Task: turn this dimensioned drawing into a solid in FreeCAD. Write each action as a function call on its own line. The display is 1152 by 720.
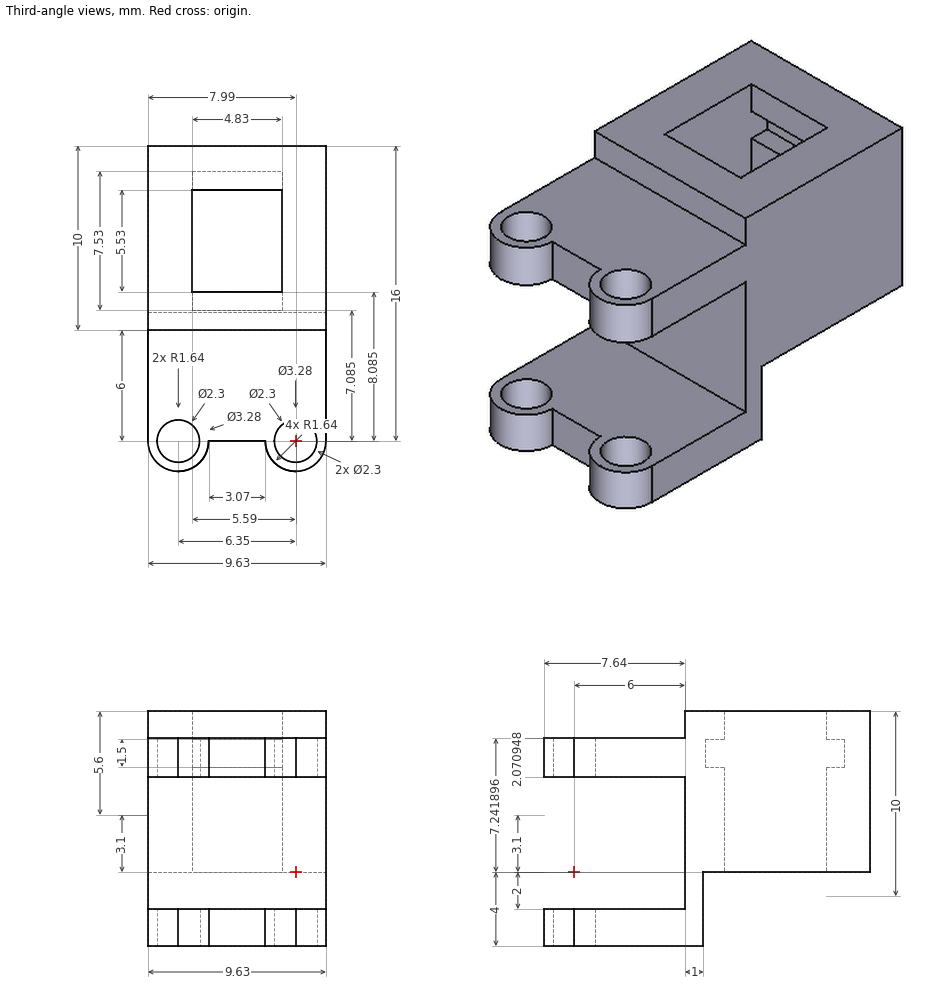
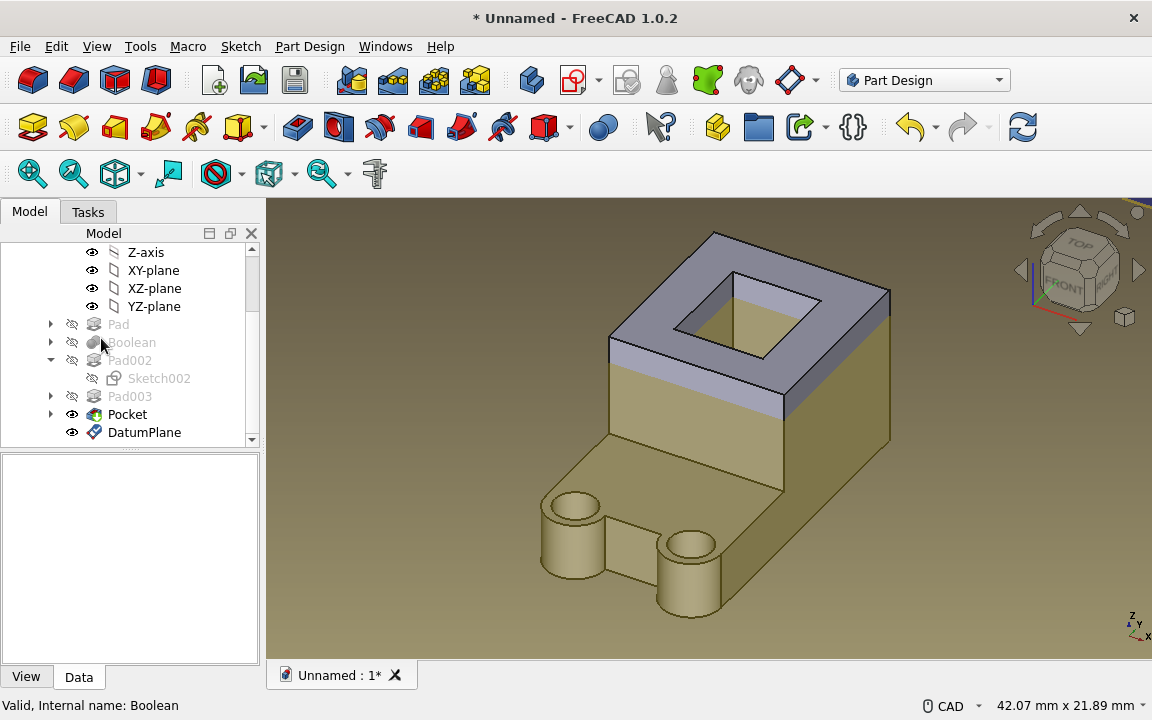
click(117, 432)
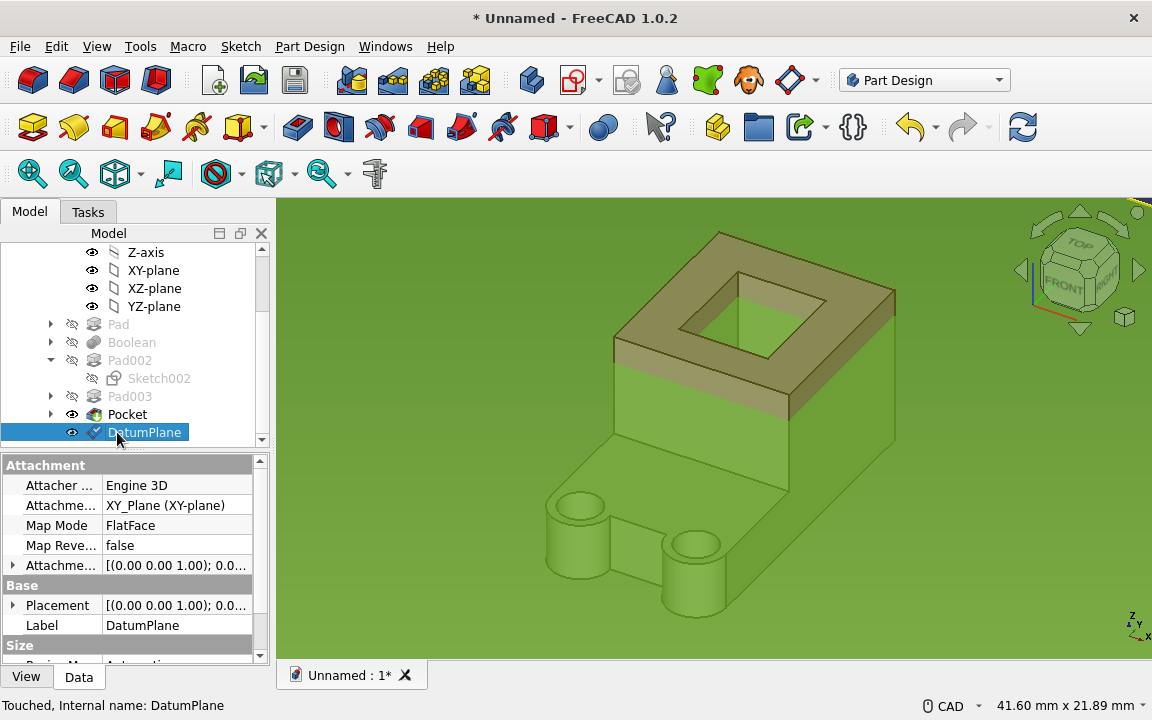
click(572, 80)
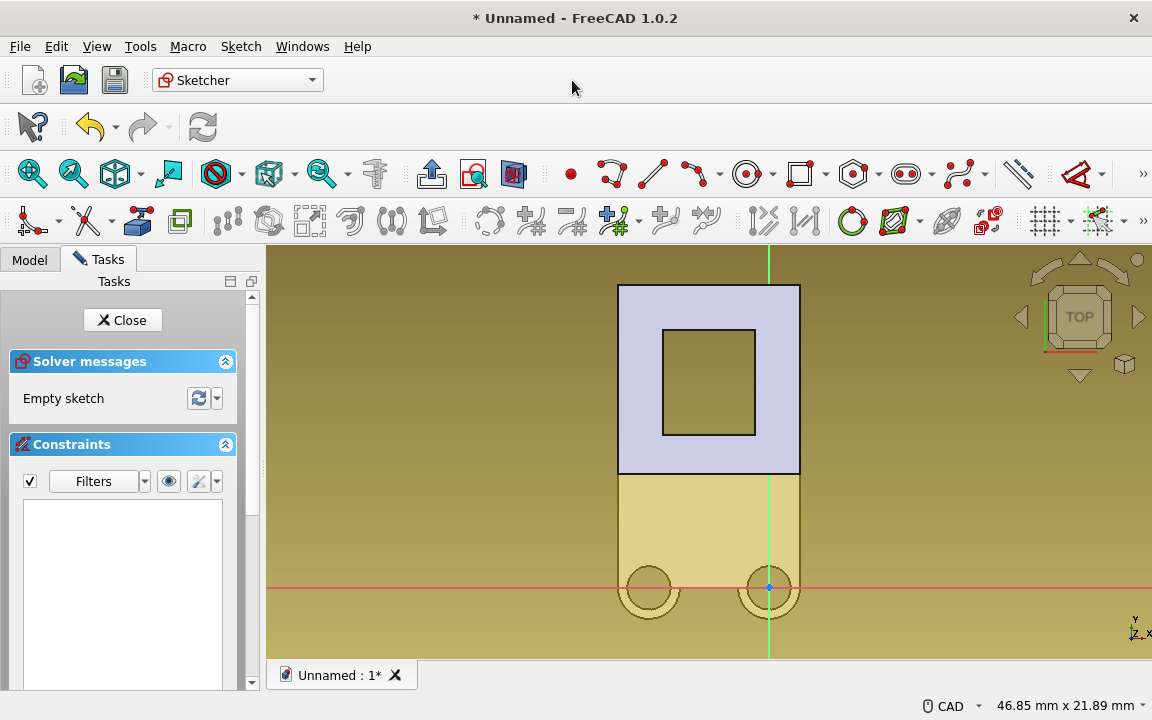
click(514, 174)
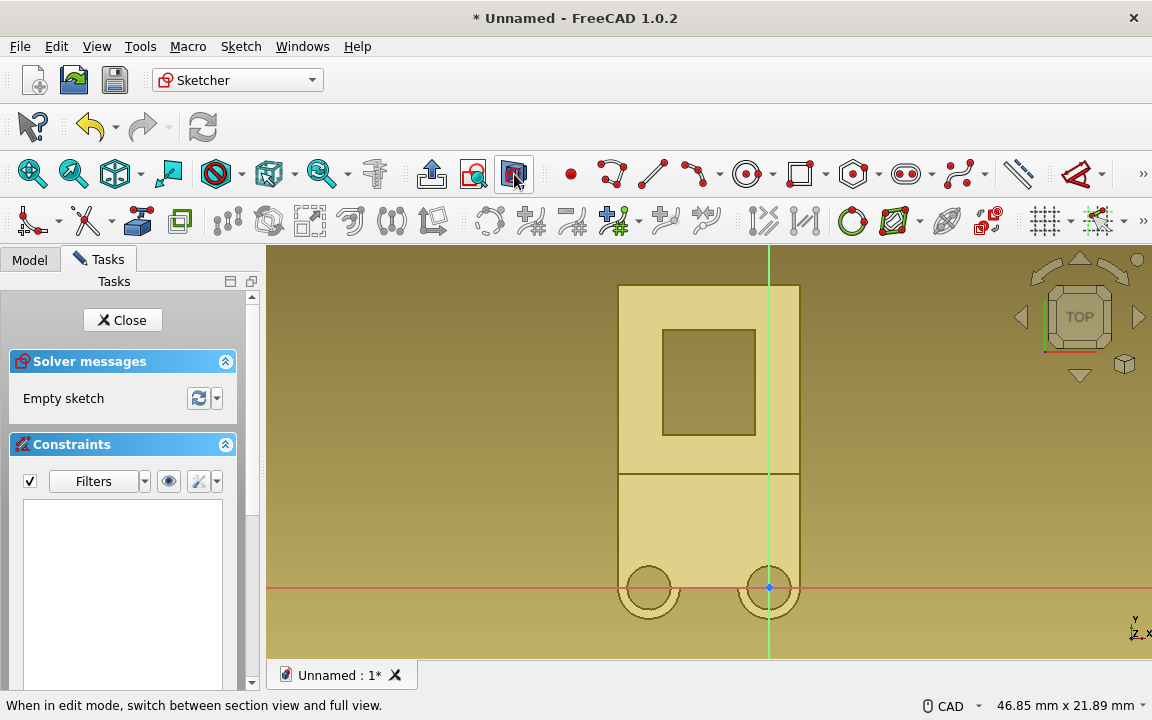
key(g)
key(r)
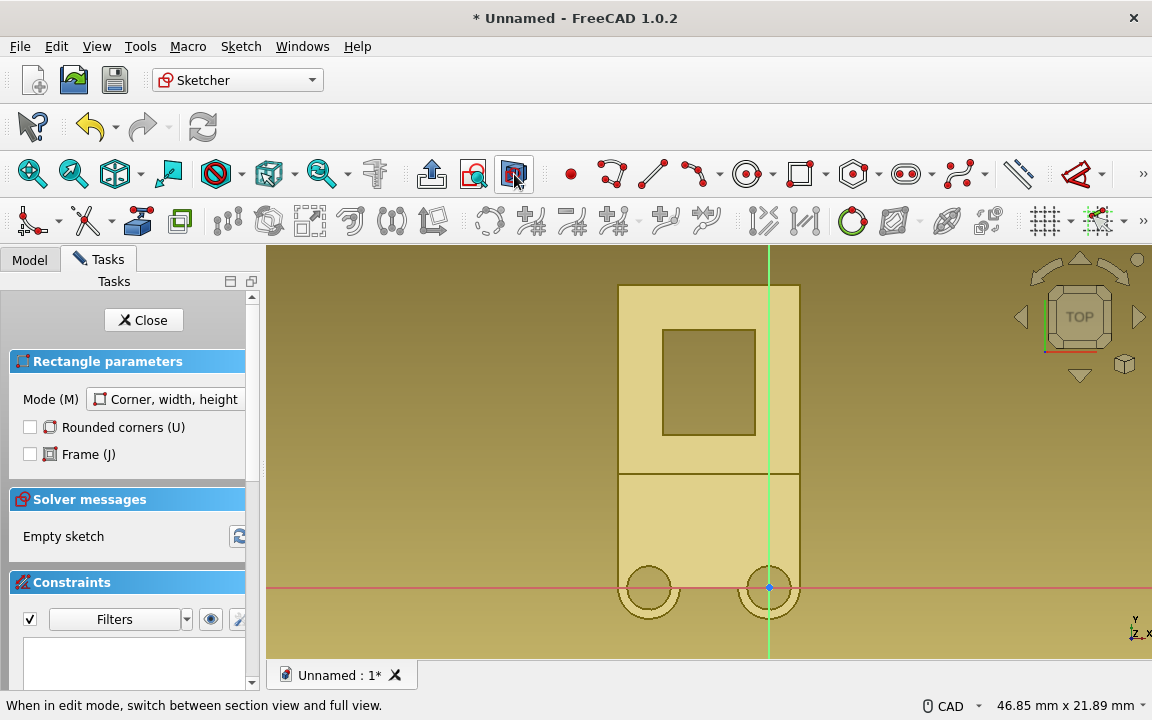
click(663, 311)
click(755, 454)
key(Escape)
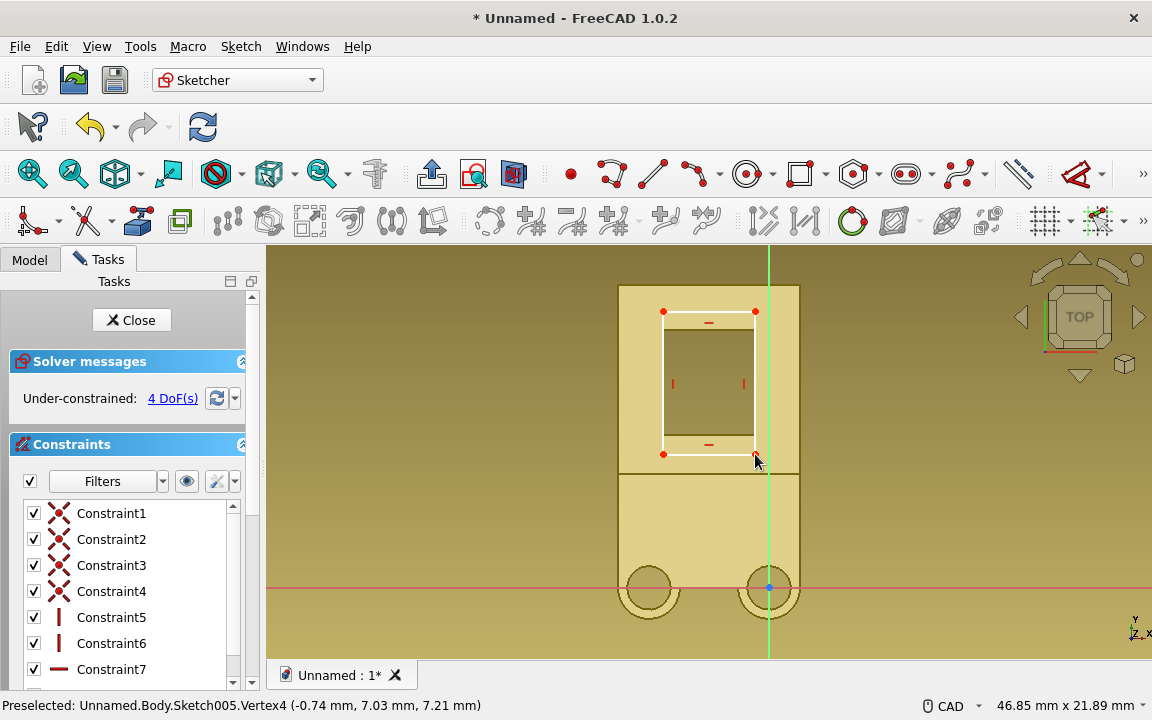
click(1076, 174)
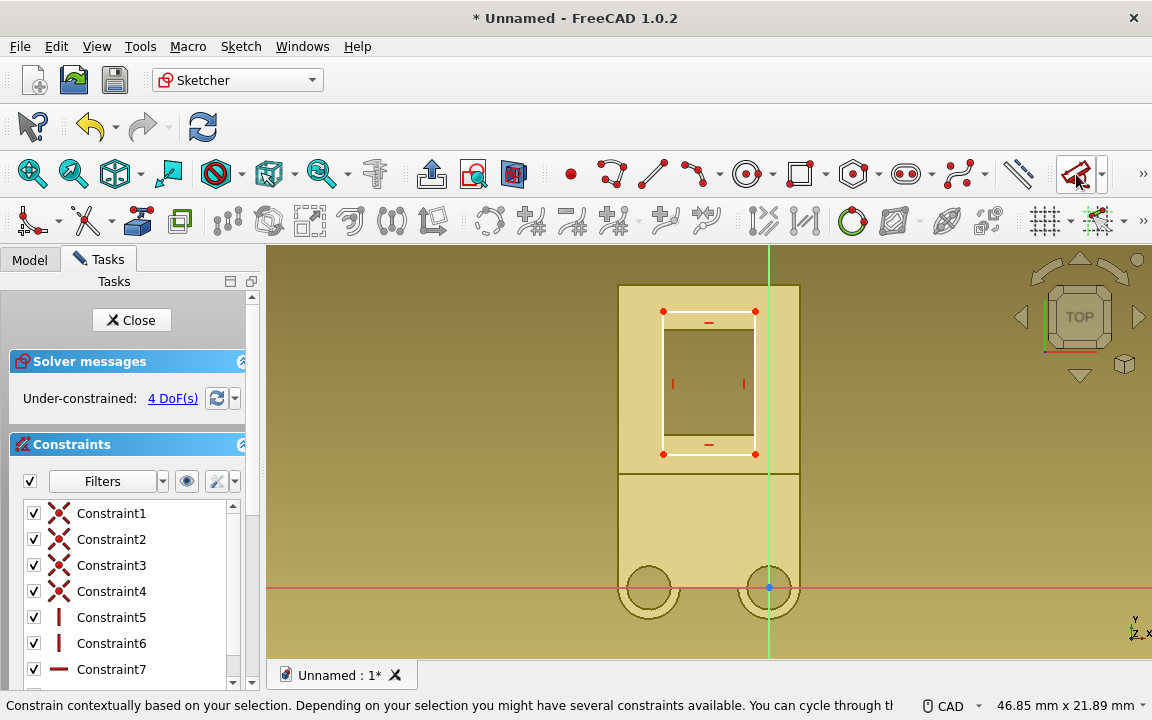
click(663, 355)
click(629, 384)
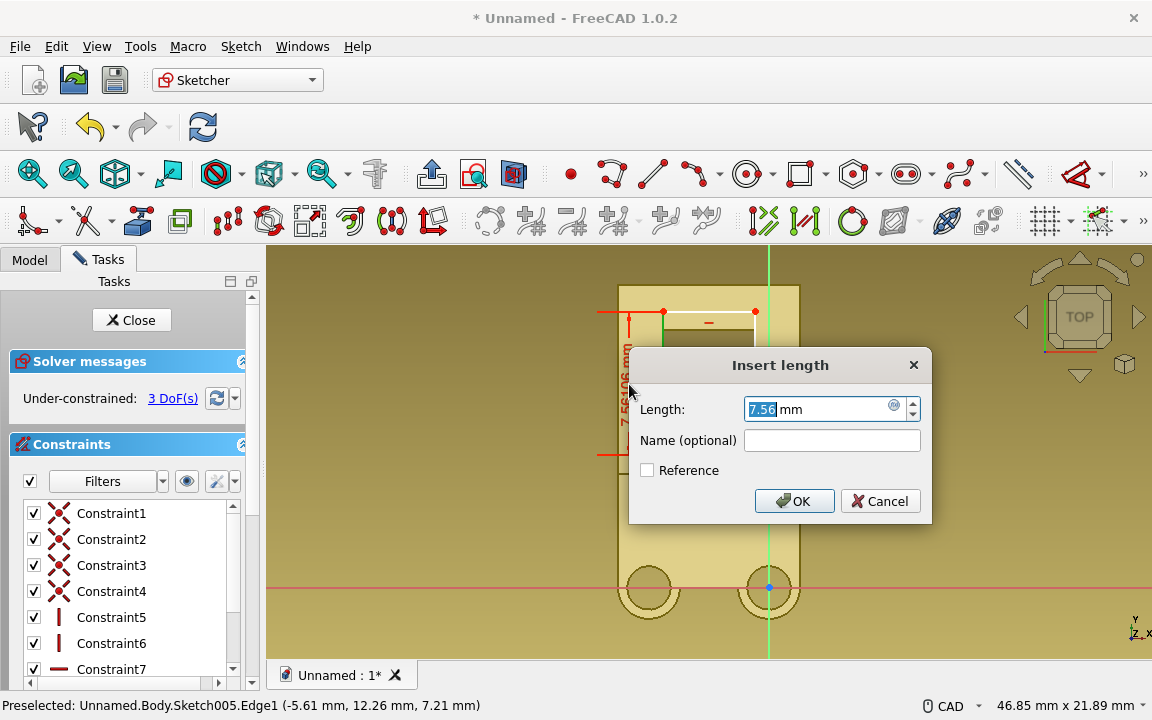
text(7.53)
key(Return)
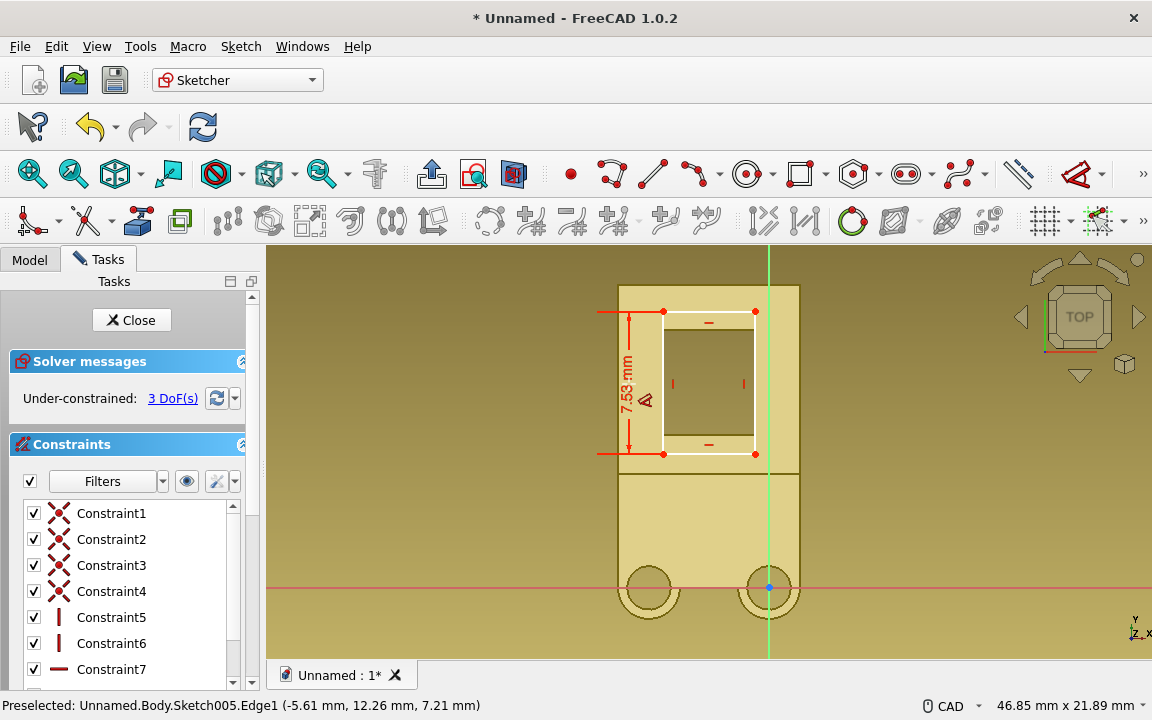
click(691, 454)
click(709, 488)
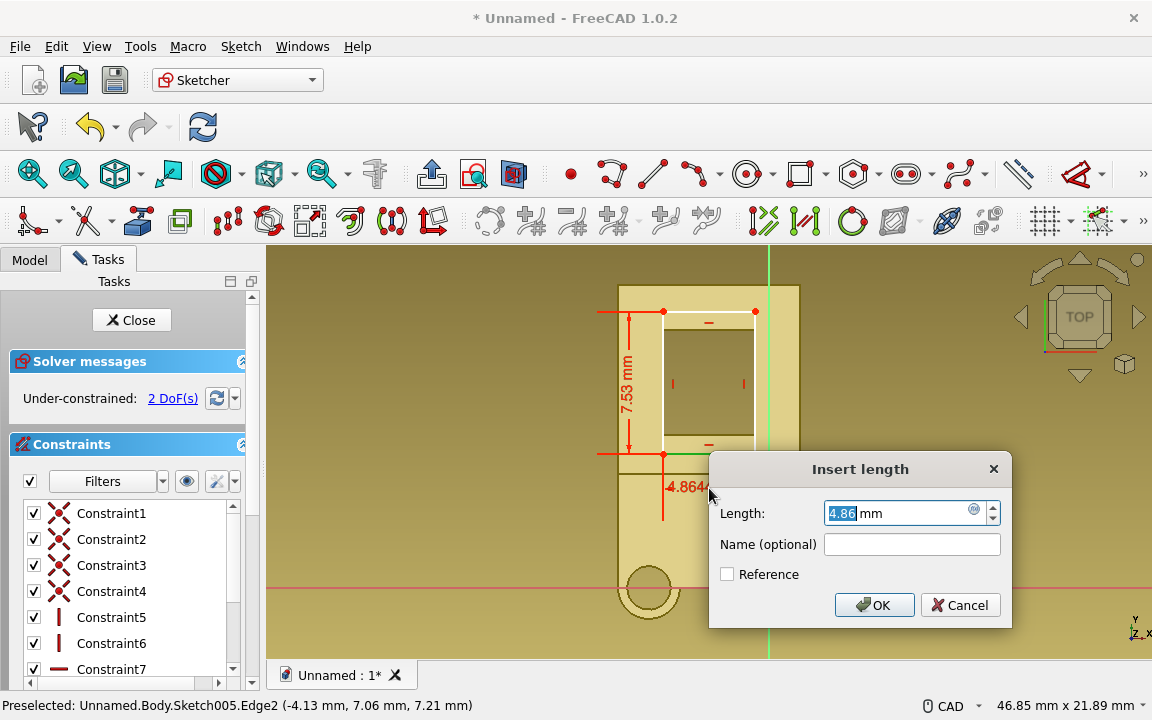
text(4.83)
key(Return)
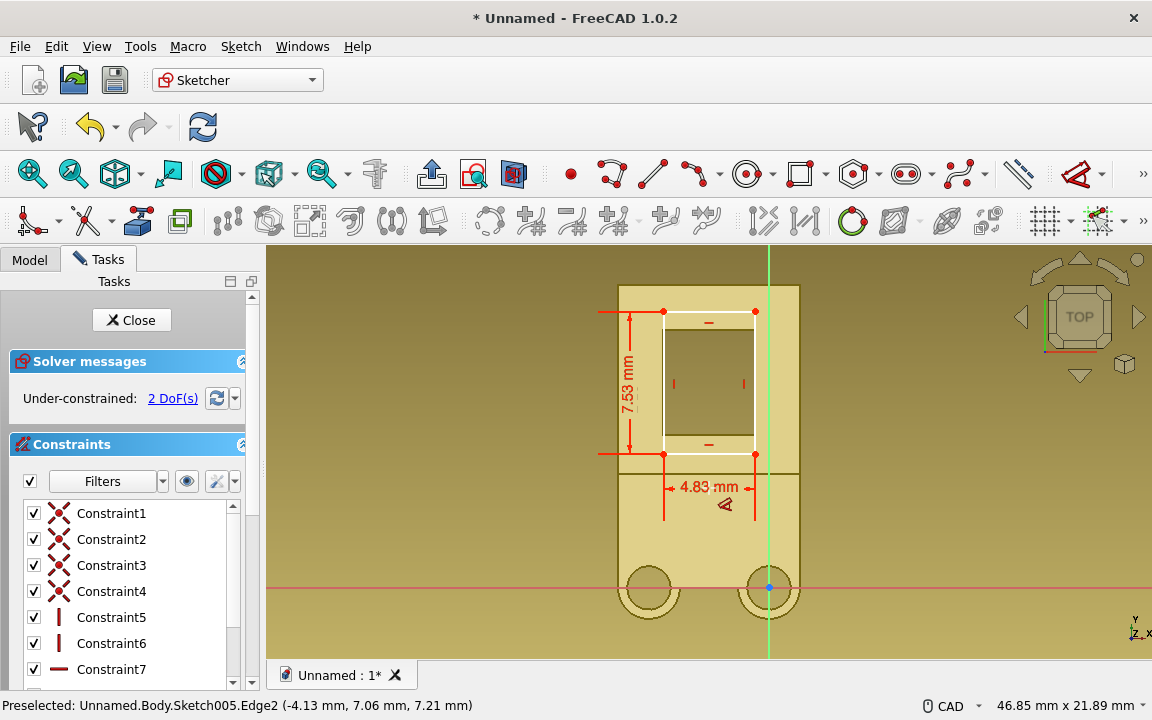
click(664, 312)
click(716, 622)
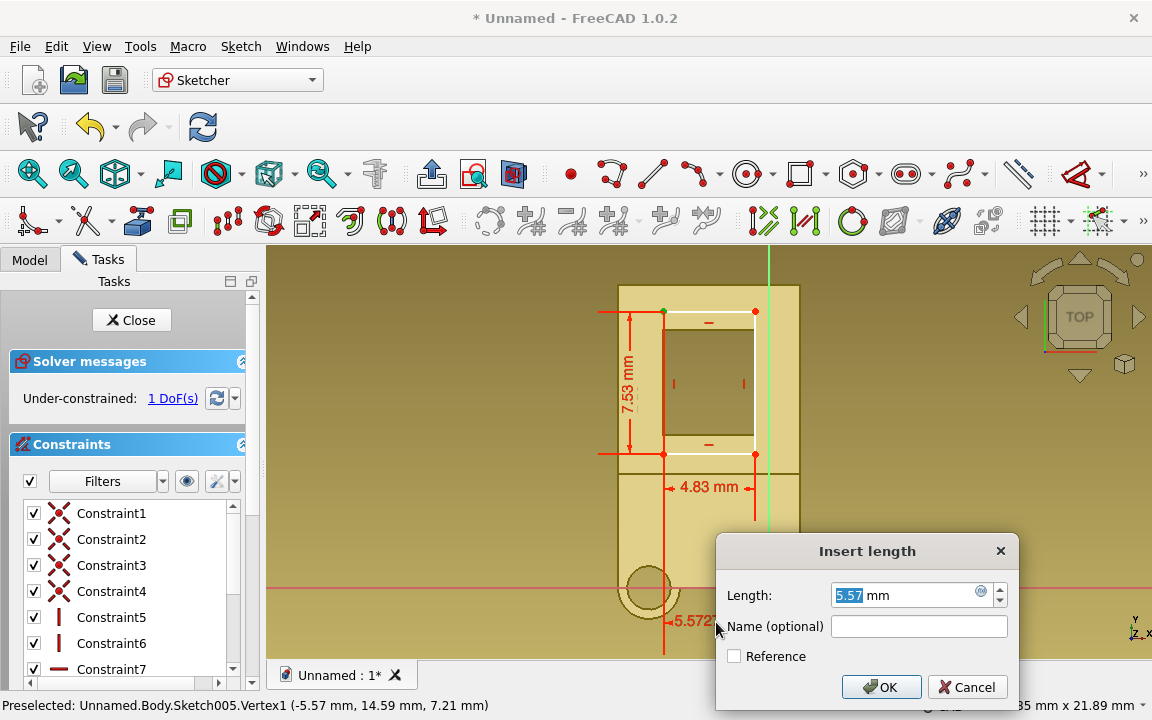
text(5.59)
key(Return)